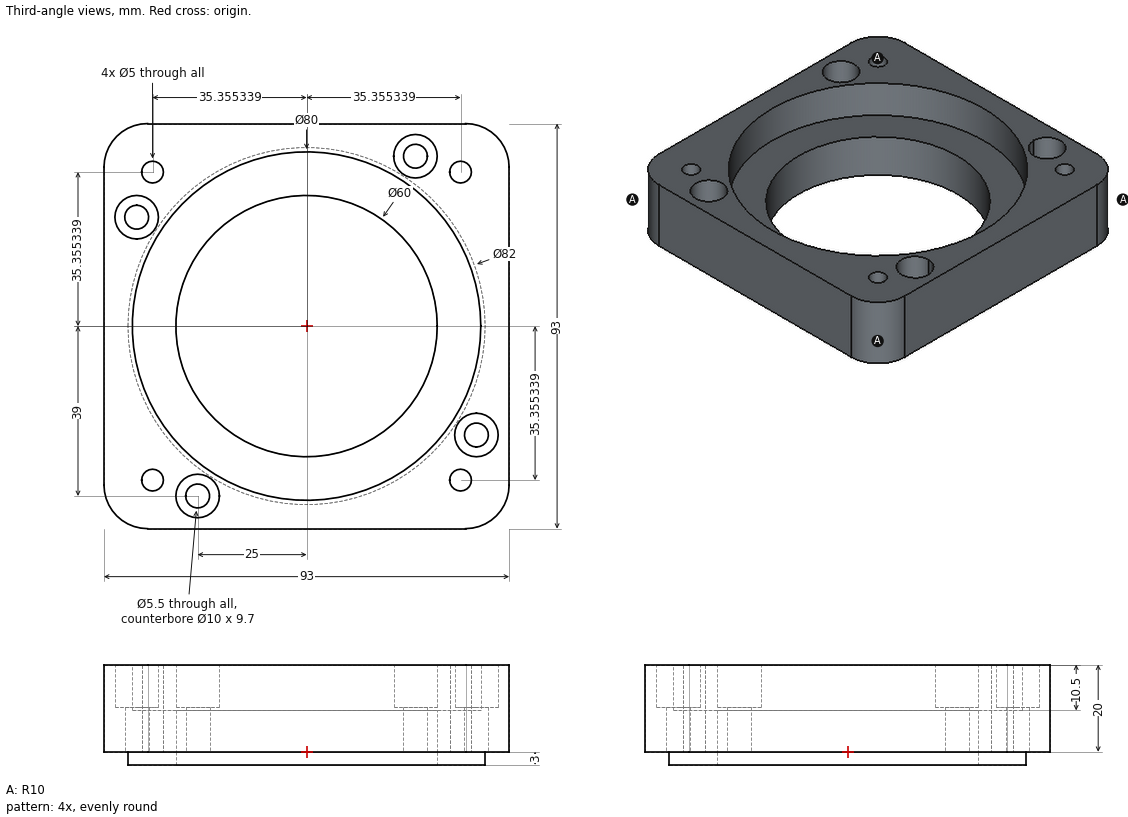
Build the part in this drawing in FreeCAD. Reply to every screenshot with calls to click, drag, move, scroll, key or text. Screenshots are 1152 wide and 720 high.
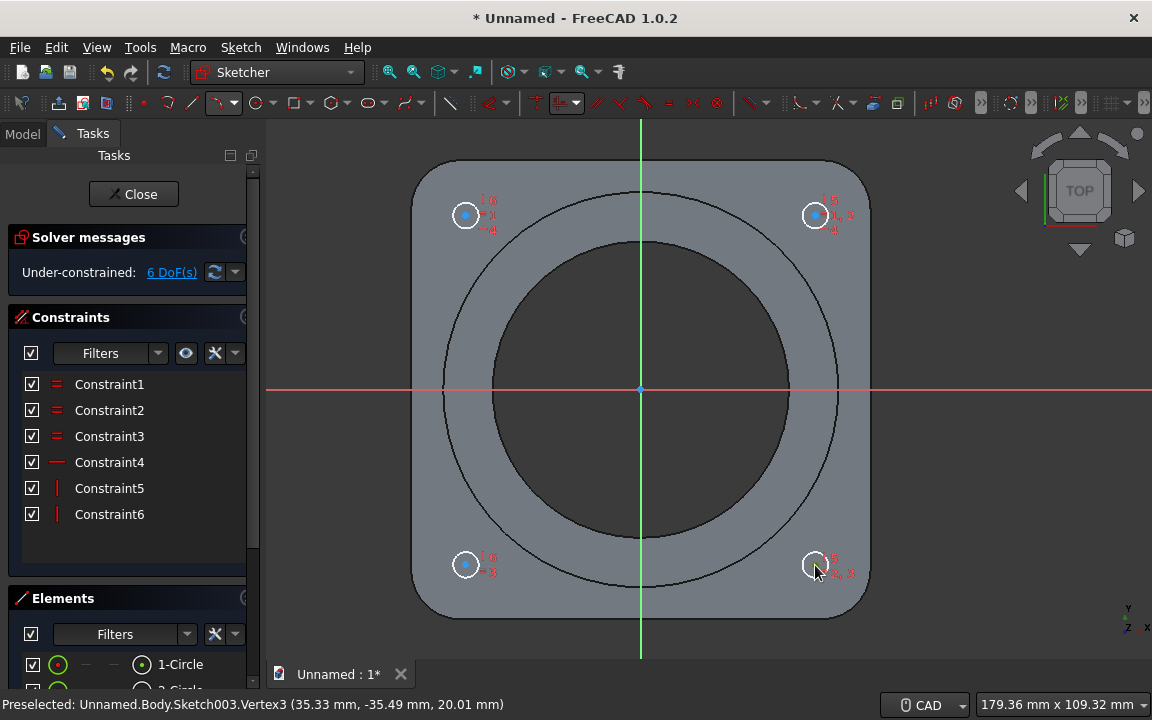
click(466, 565)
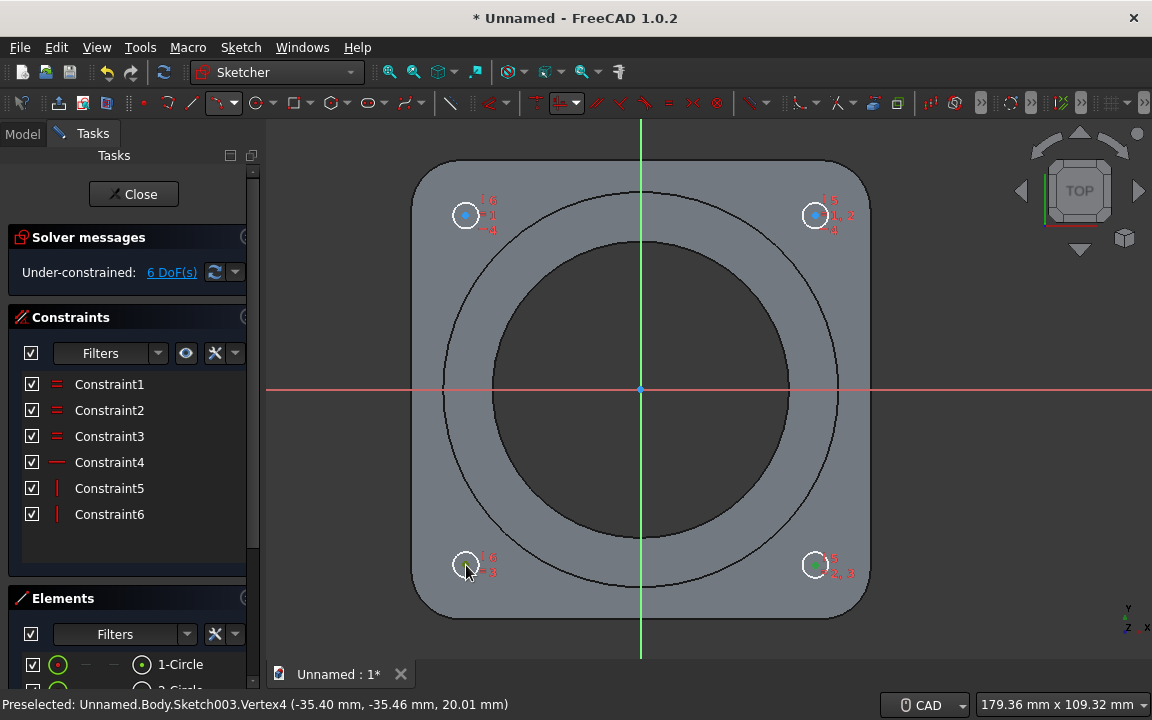
click(578, 104)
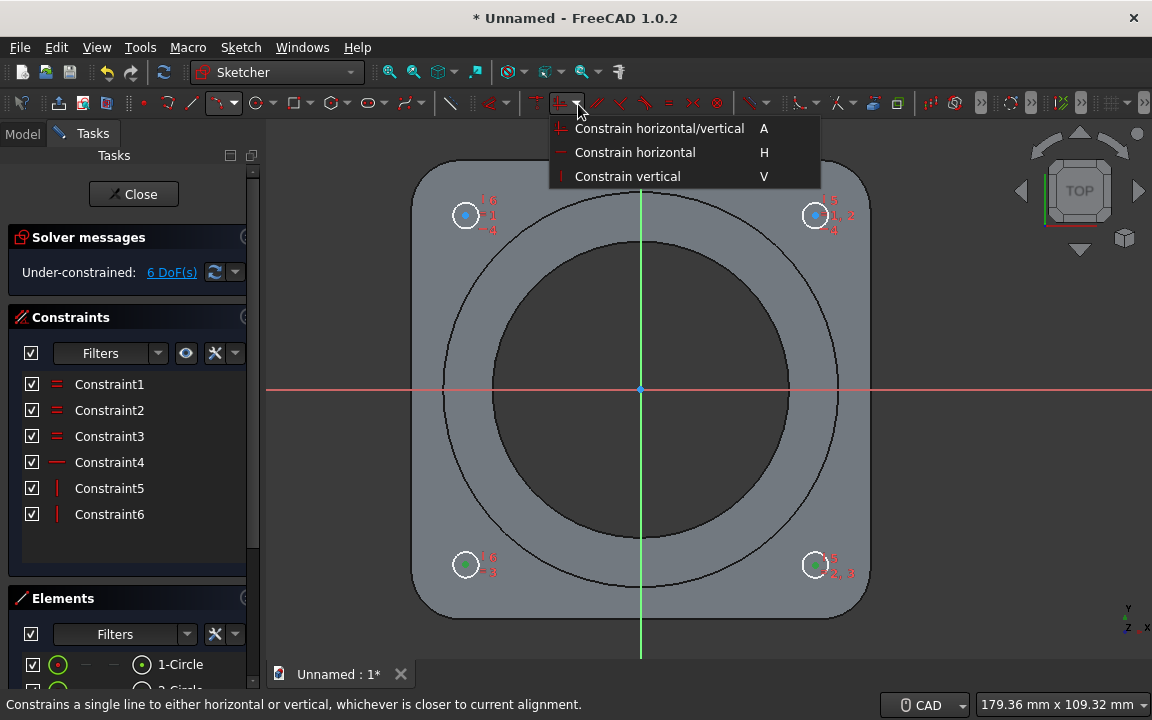
click(685, 152)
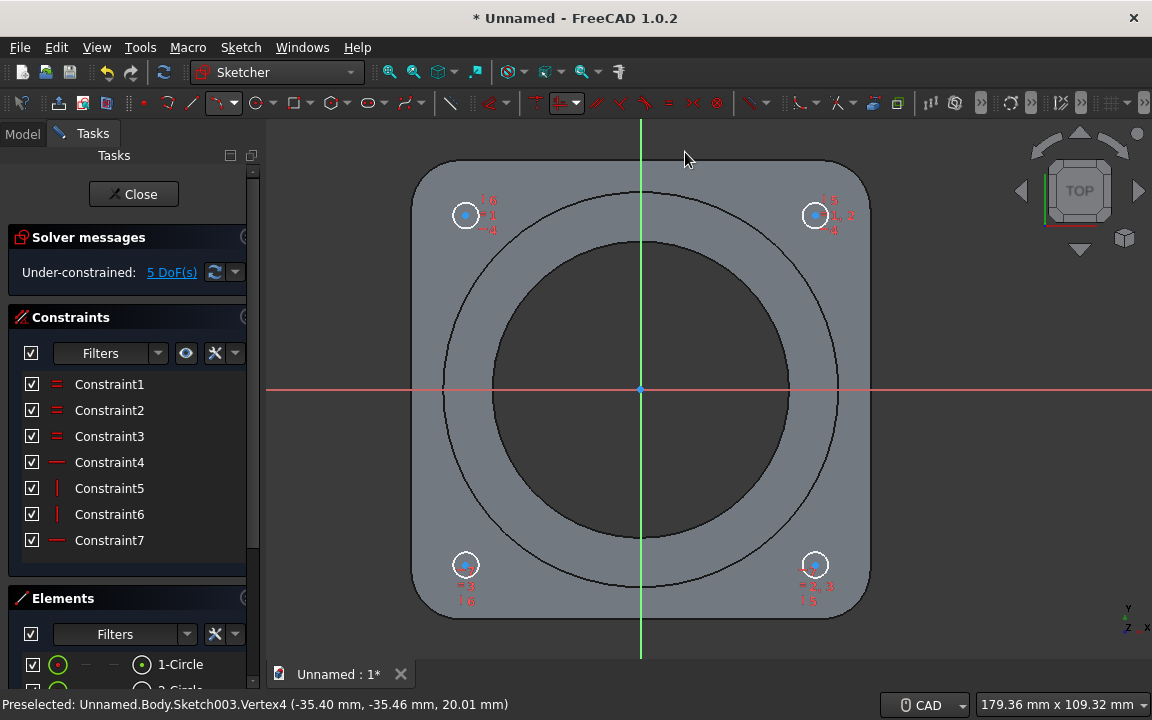
click(490, 104)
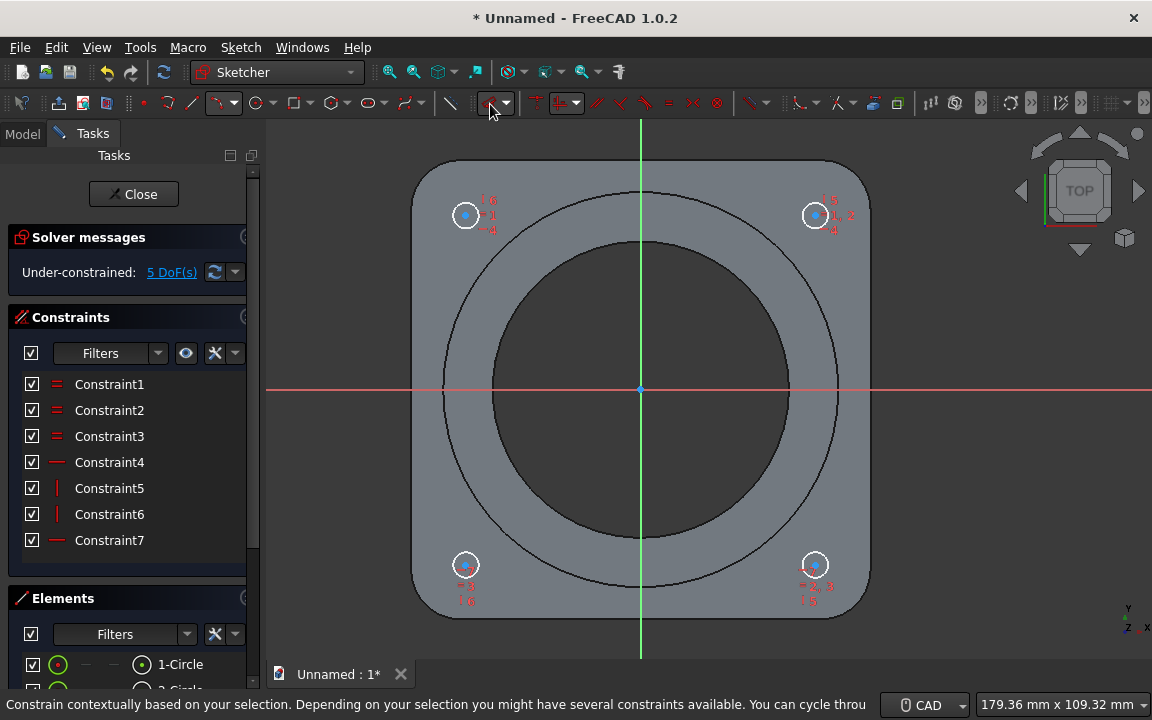
scroll(475, 207, up, 3)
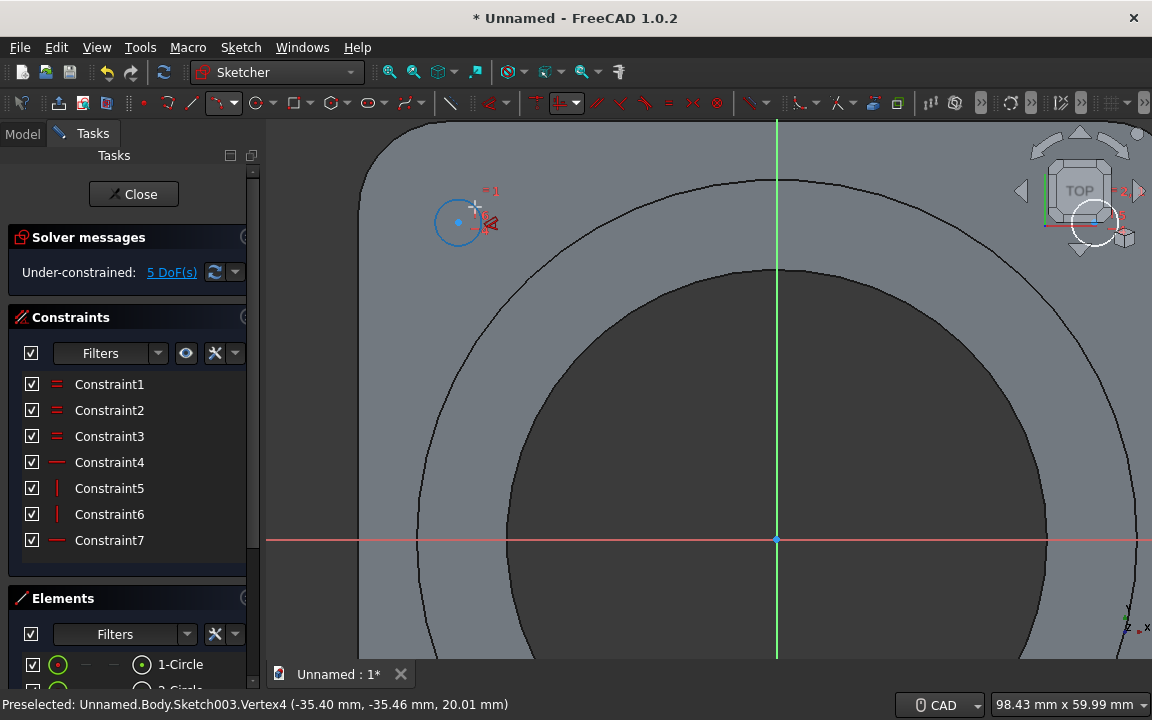
click(475, 206)
click(498, 183)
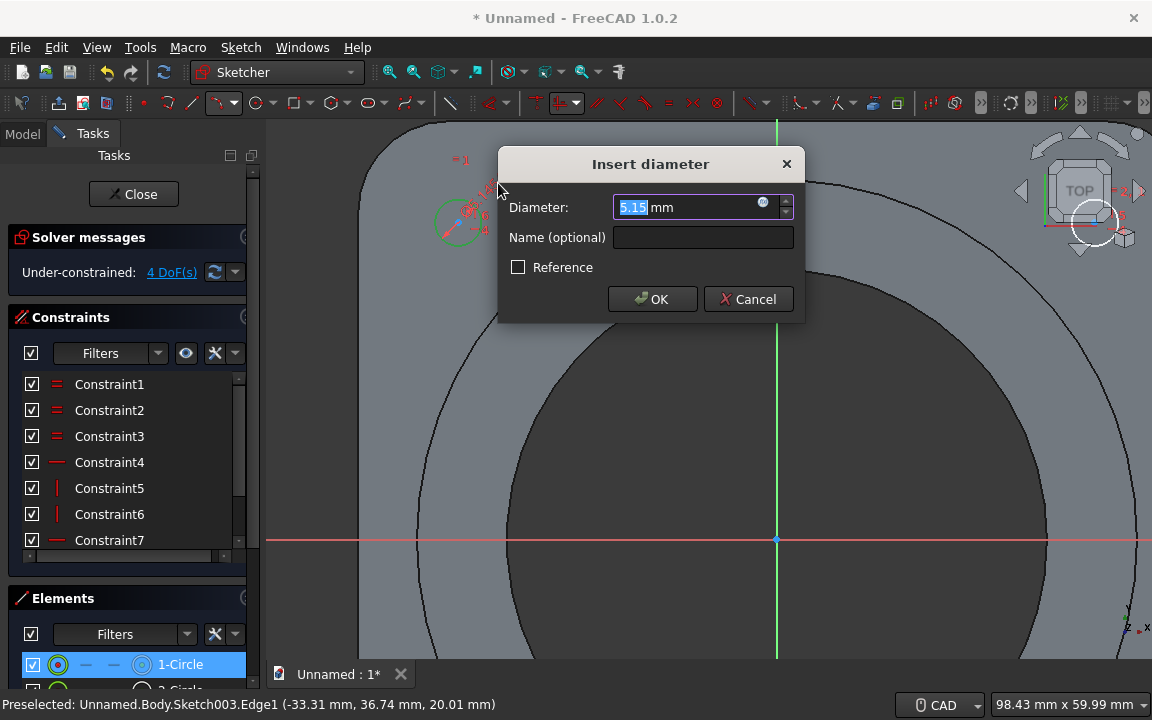
text(5)
key(Return)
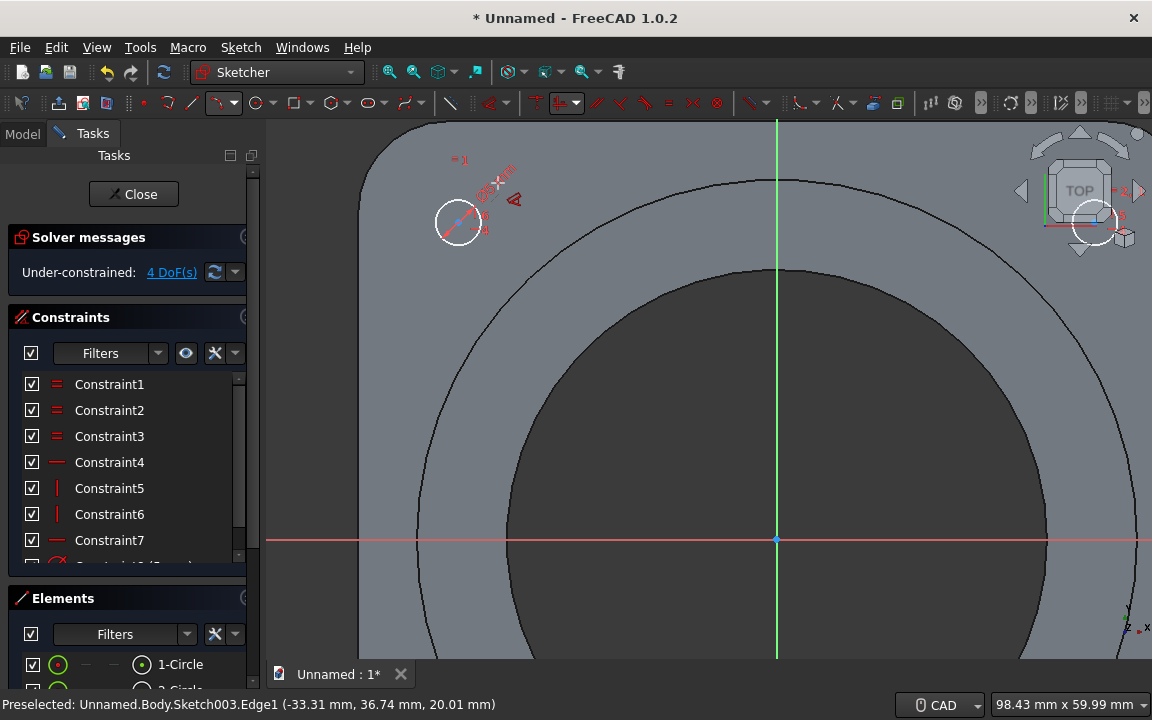
click(458, 223)
click(618, 189)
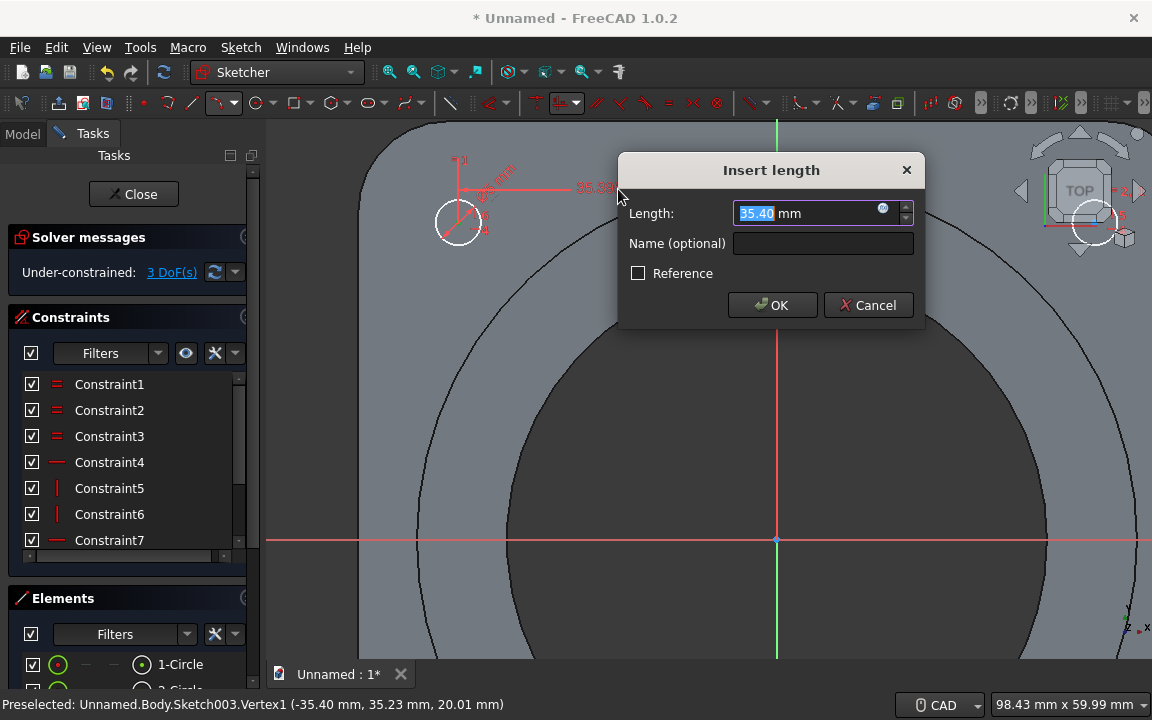
text(35.355339)
key(Return)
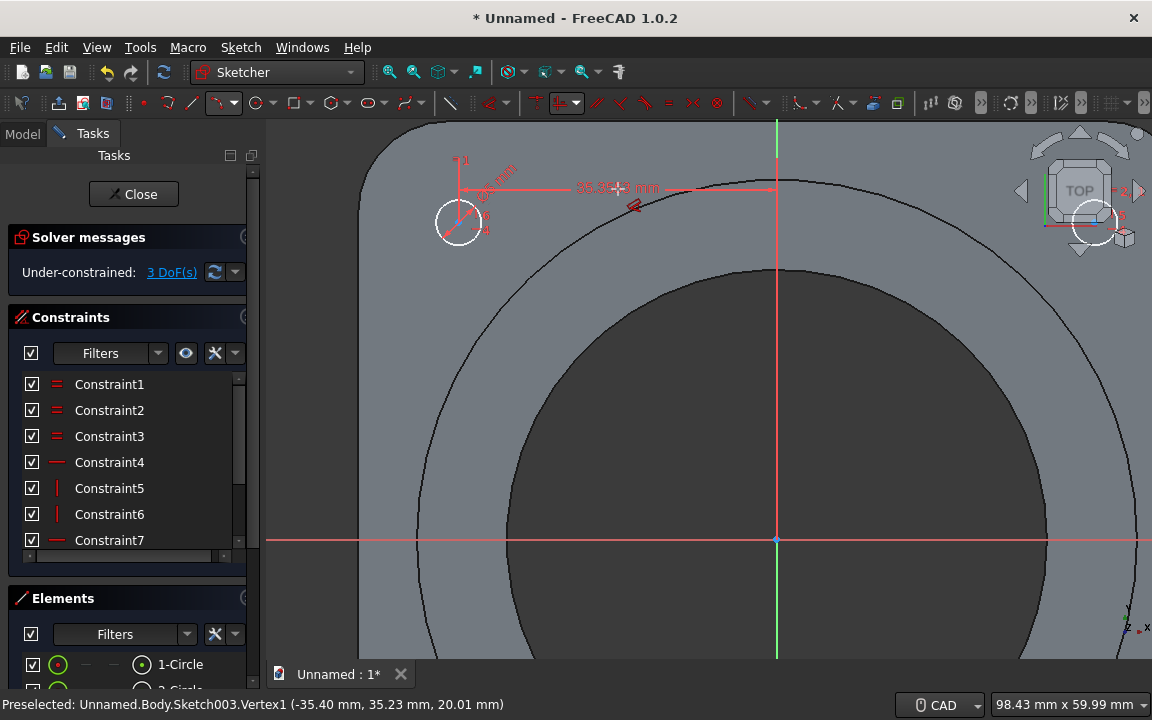
click(459, 223)
click(425, 381)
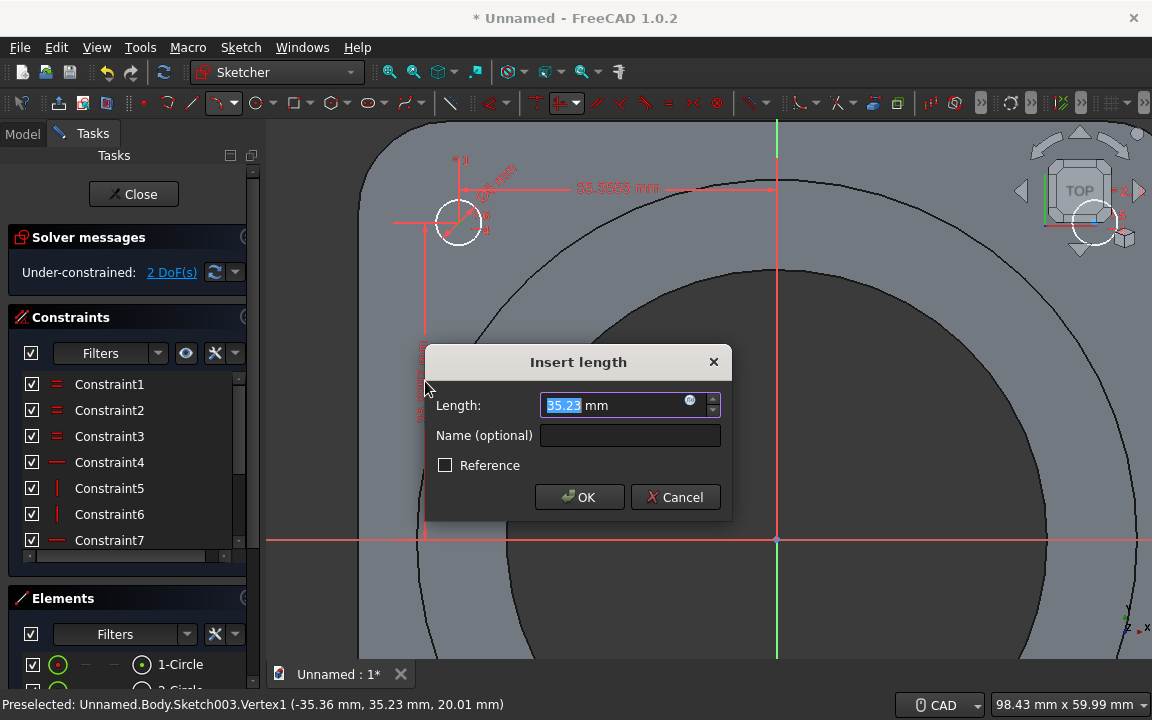
text(35.355339)
key(Return)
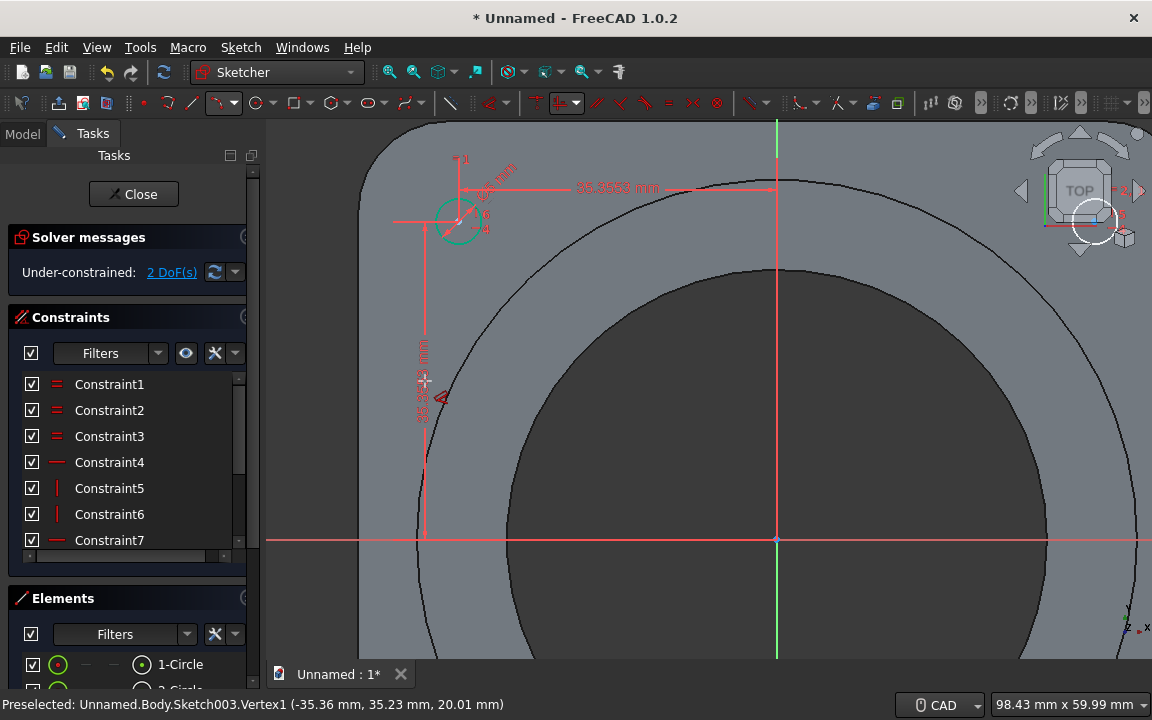
scroll(475, 206, down, 3)